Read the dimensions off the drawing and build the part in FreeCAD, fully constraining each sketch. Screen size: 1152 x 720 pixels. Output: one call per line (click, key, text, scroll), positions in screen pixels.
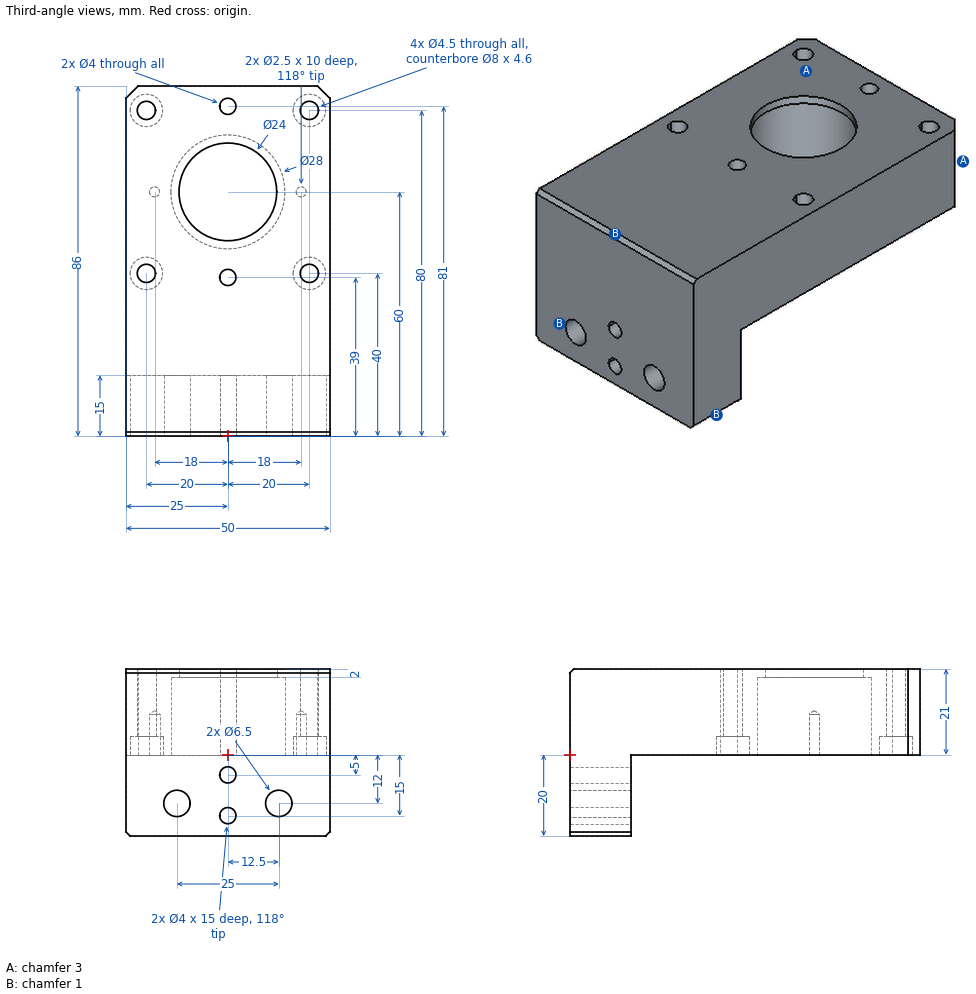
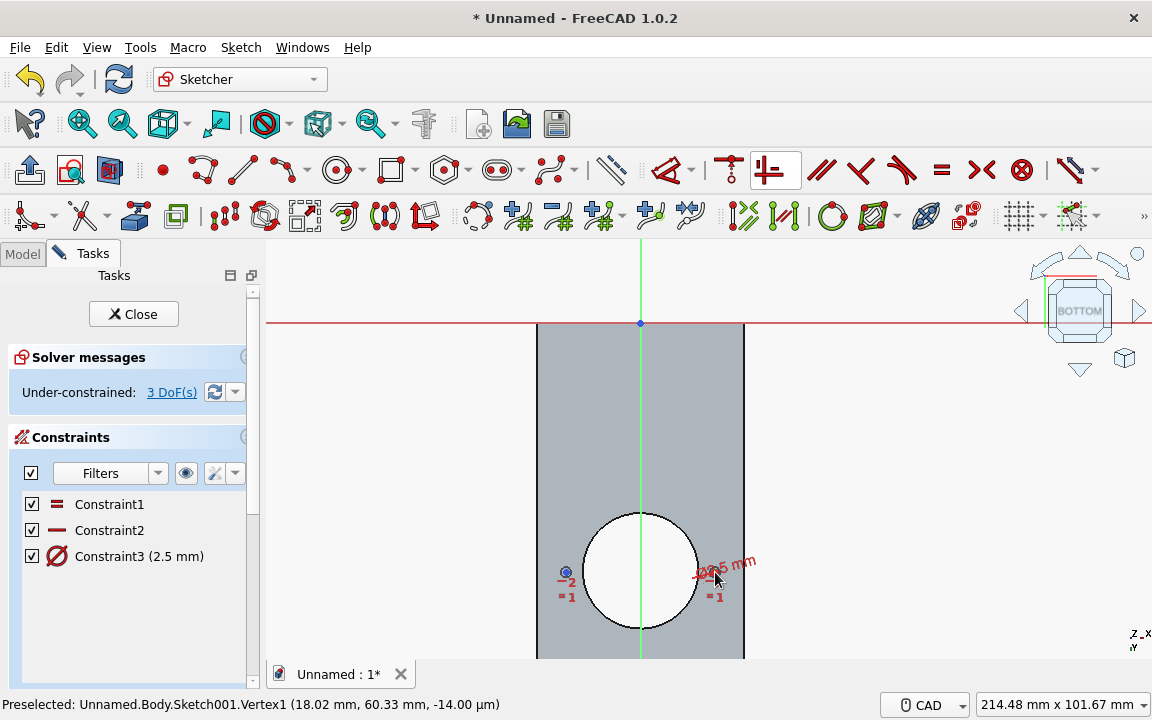
click(694, 170)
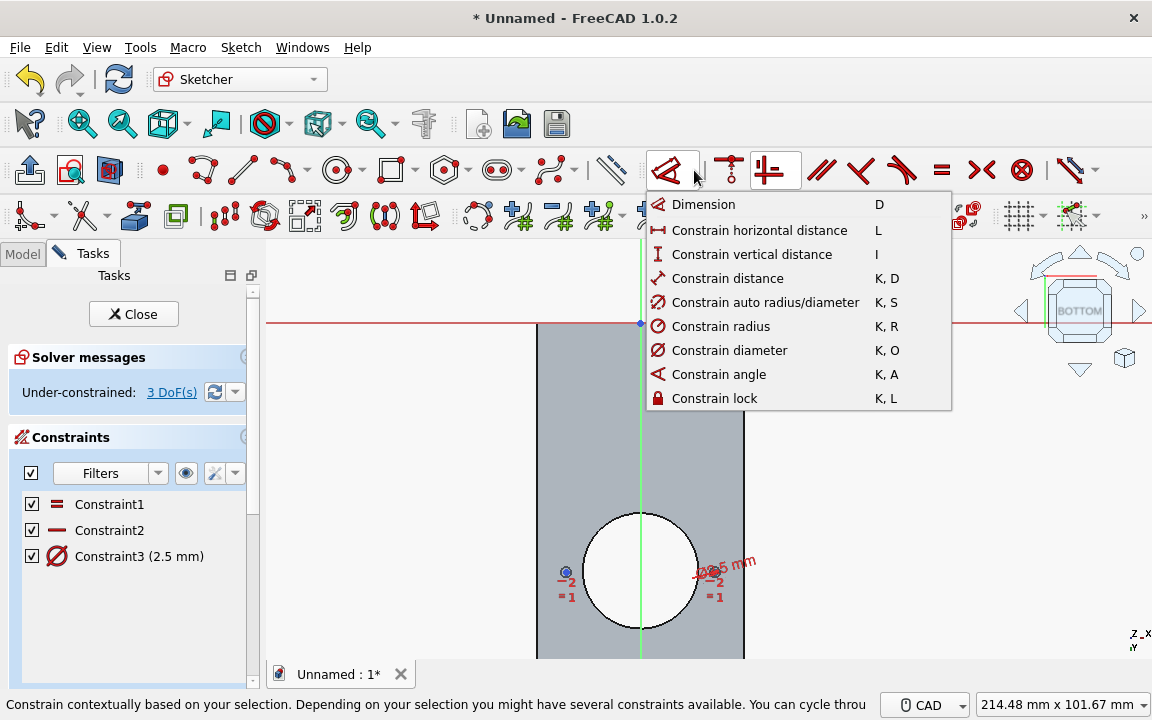
click(799, 230)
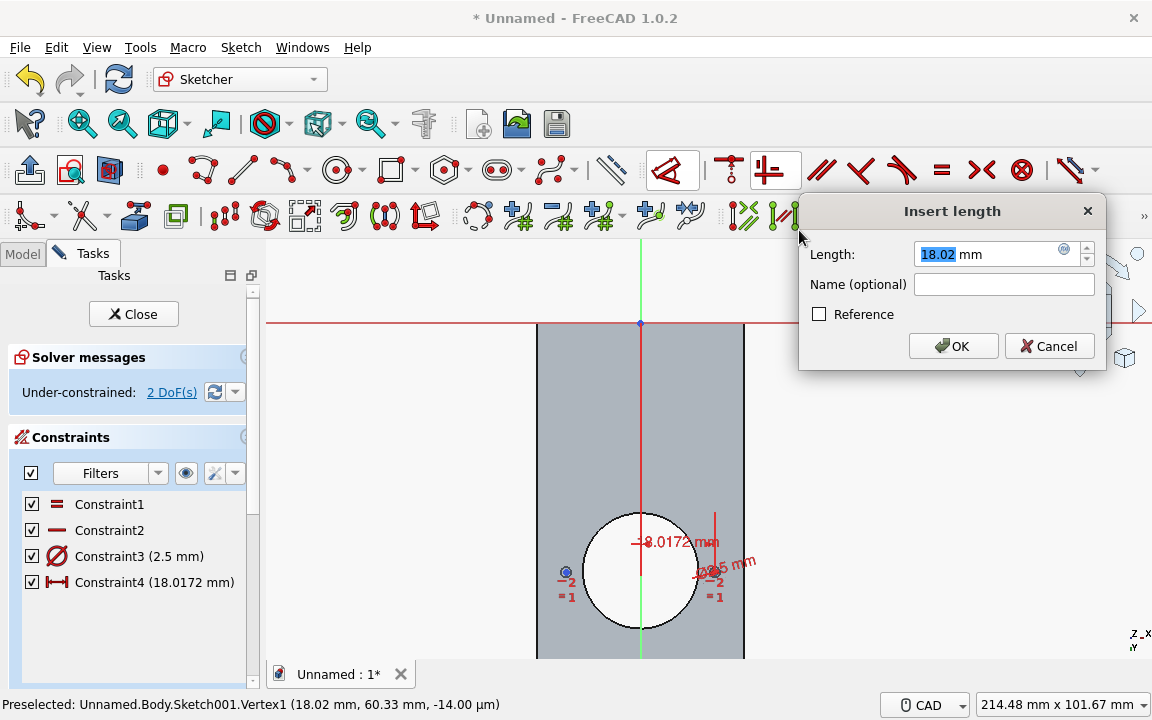
text(18)
key(Return)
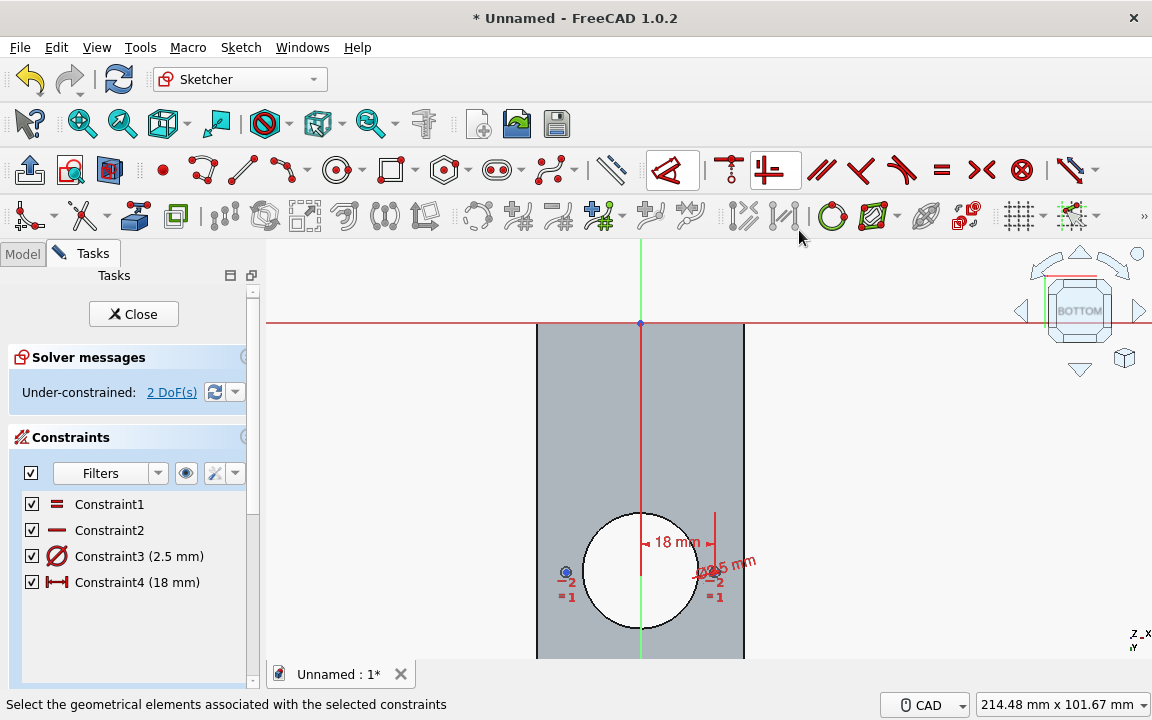
click(715, 572)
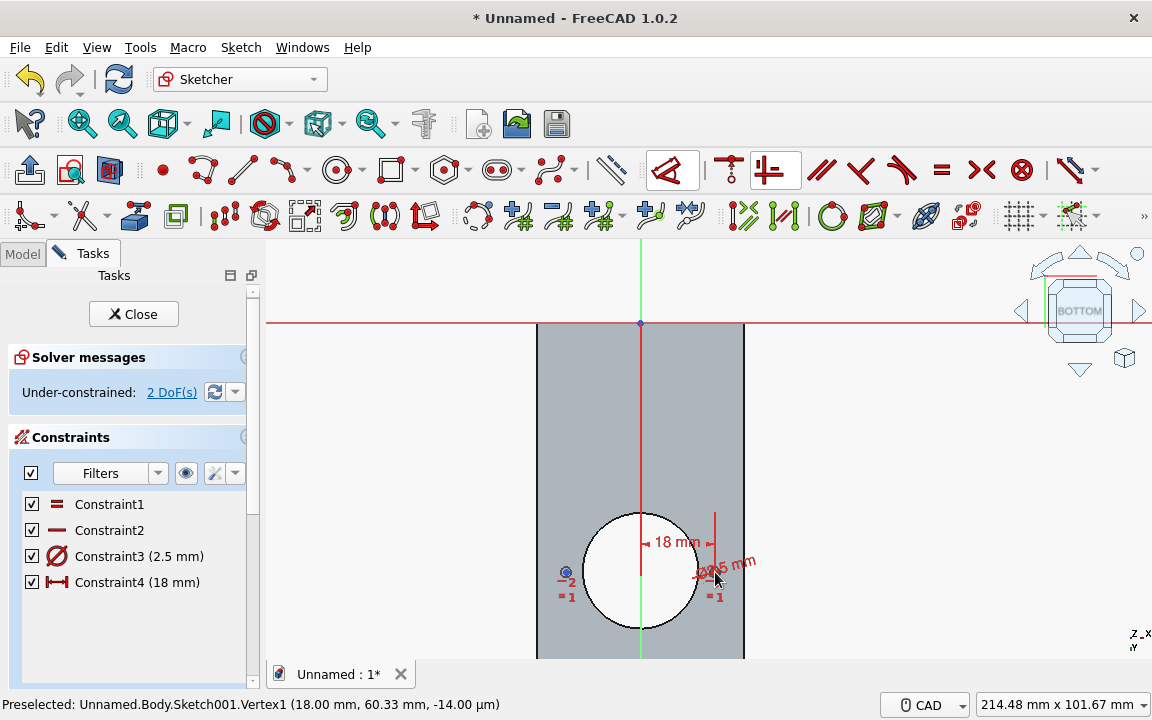
key(i)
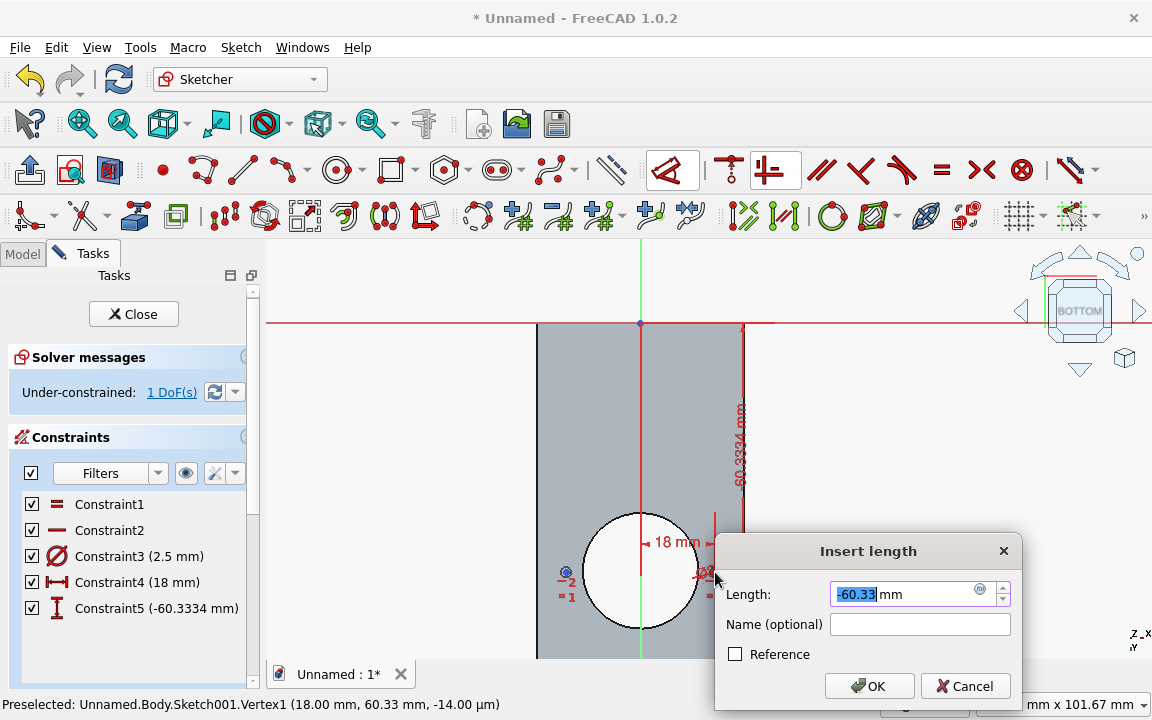
text(-60)
key(Return)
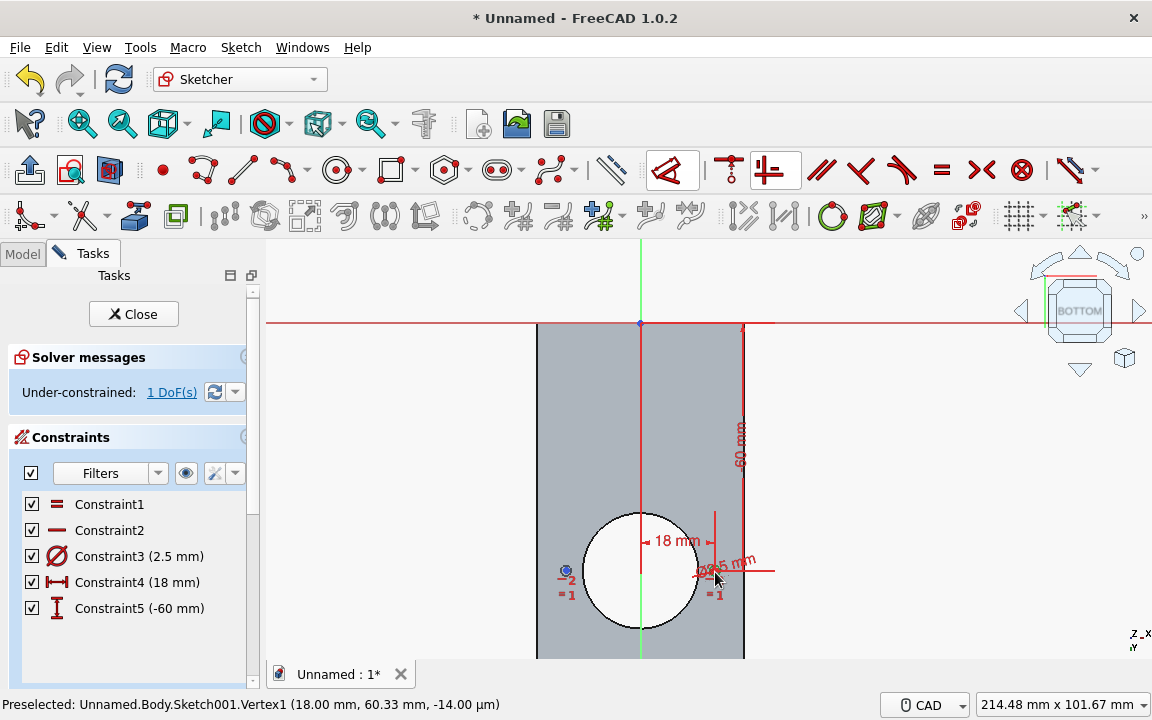
click(566, 571)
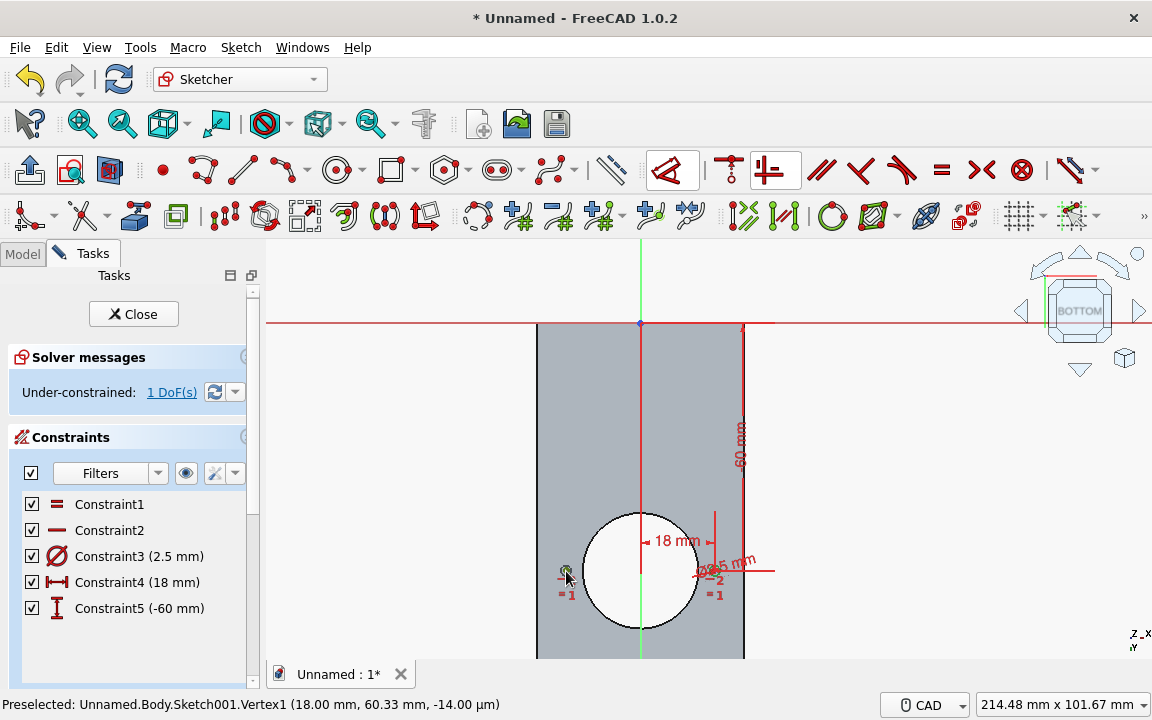
click(694, 170)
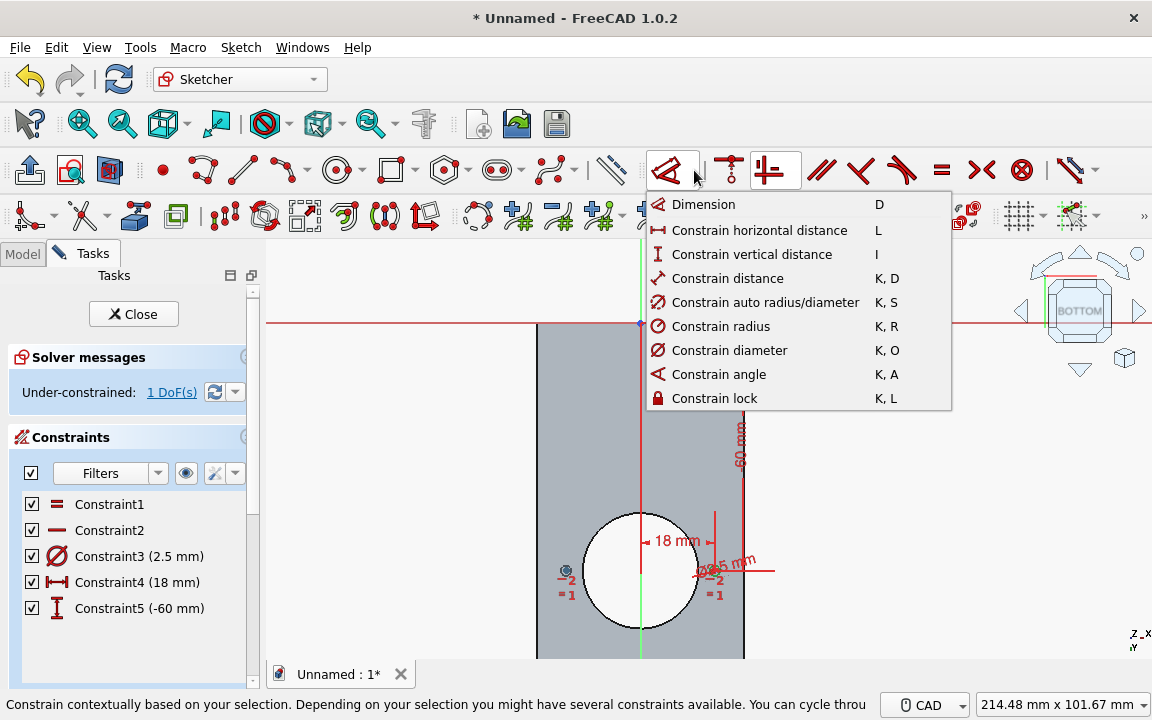
click(799, 230)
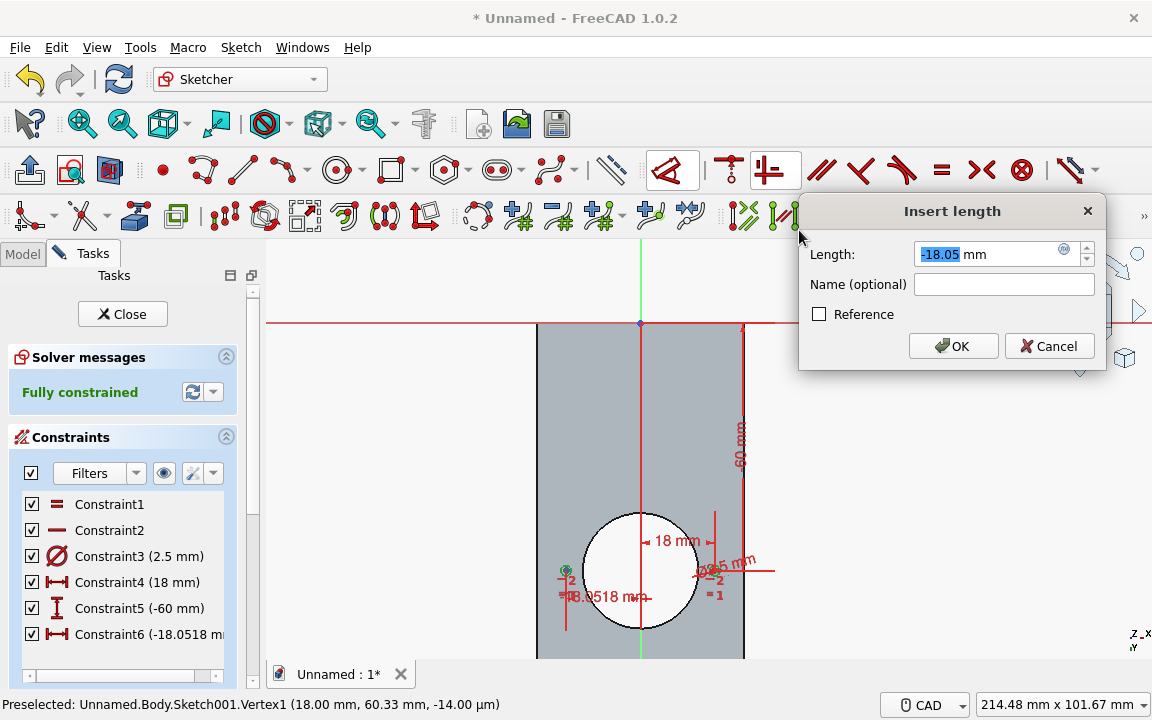
text(-18)
key(Return)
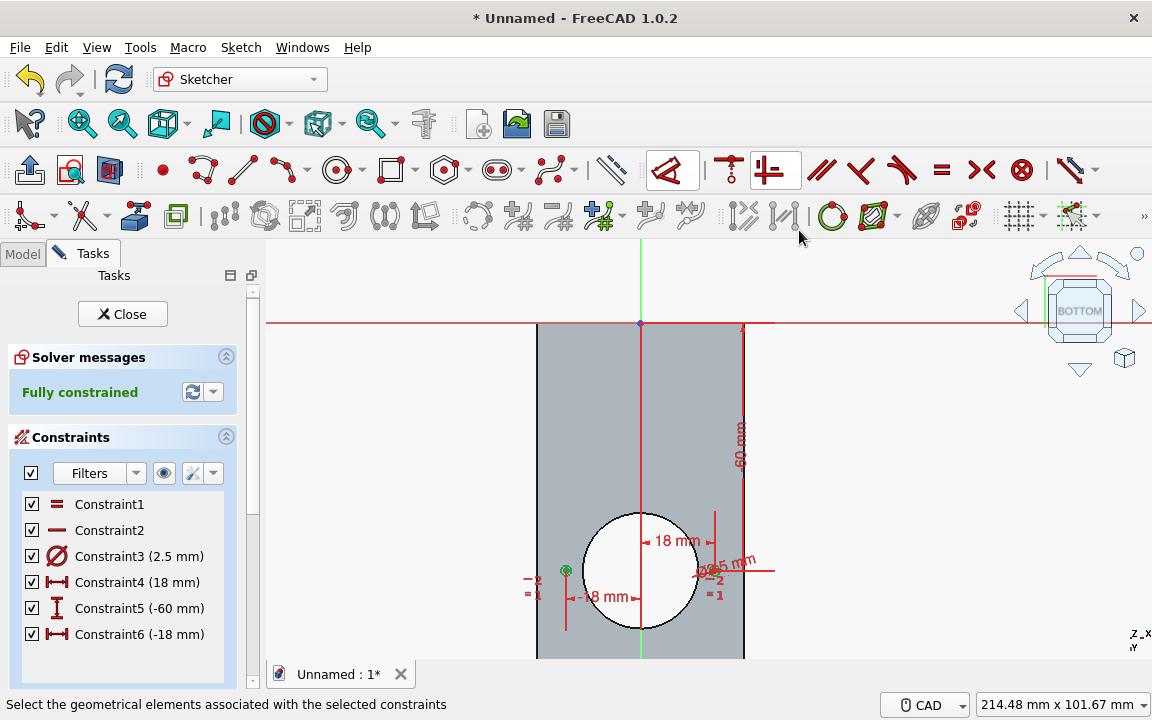
click(123, 314)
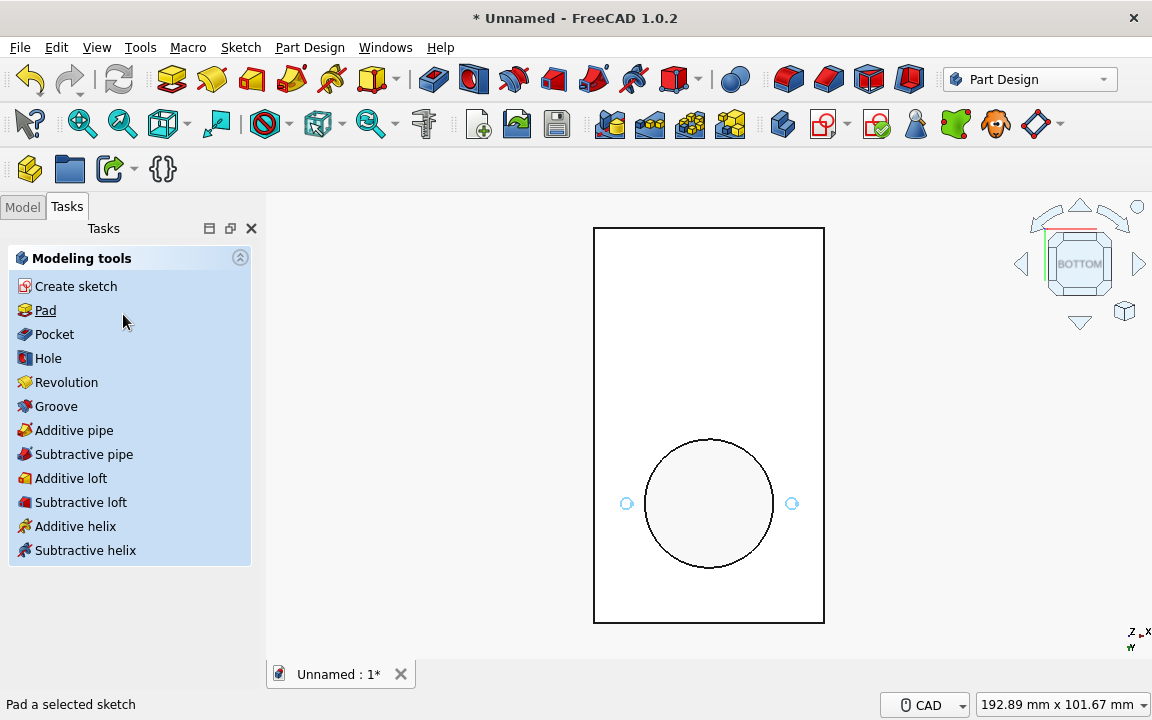
click(474, 80)